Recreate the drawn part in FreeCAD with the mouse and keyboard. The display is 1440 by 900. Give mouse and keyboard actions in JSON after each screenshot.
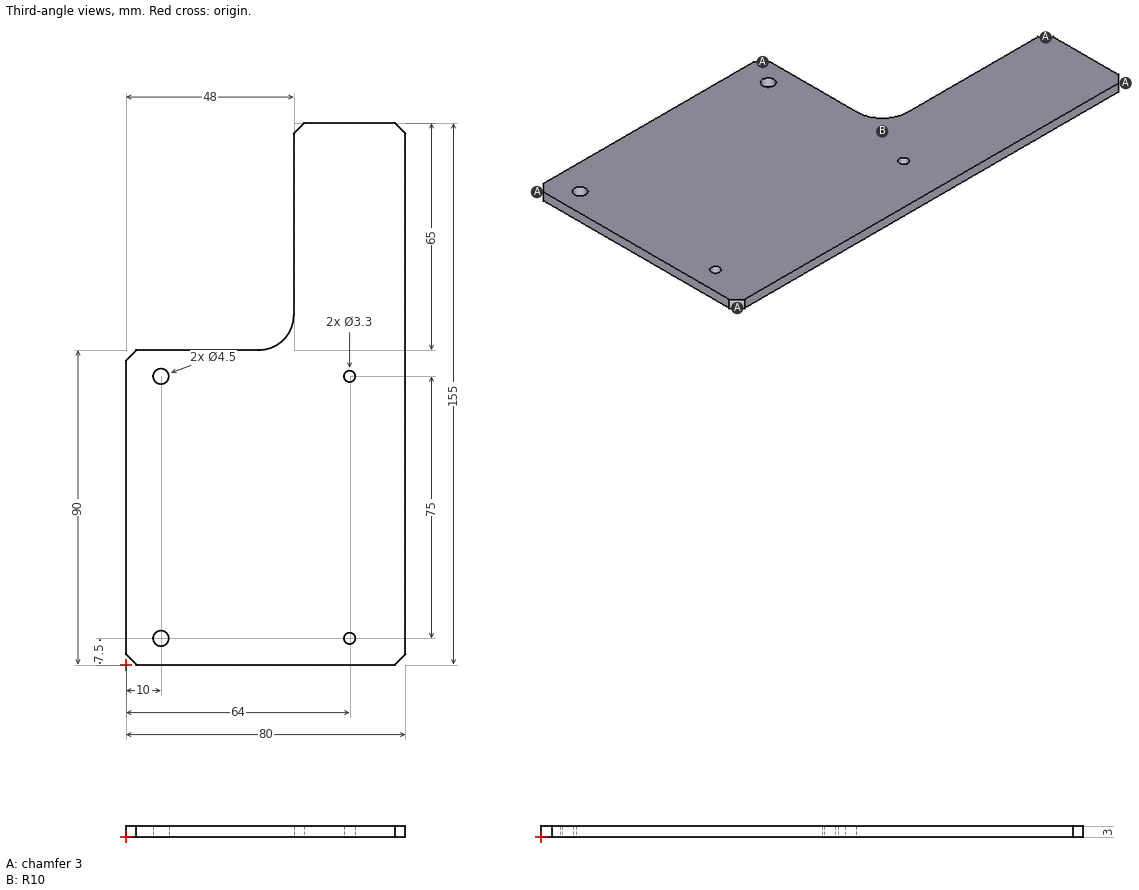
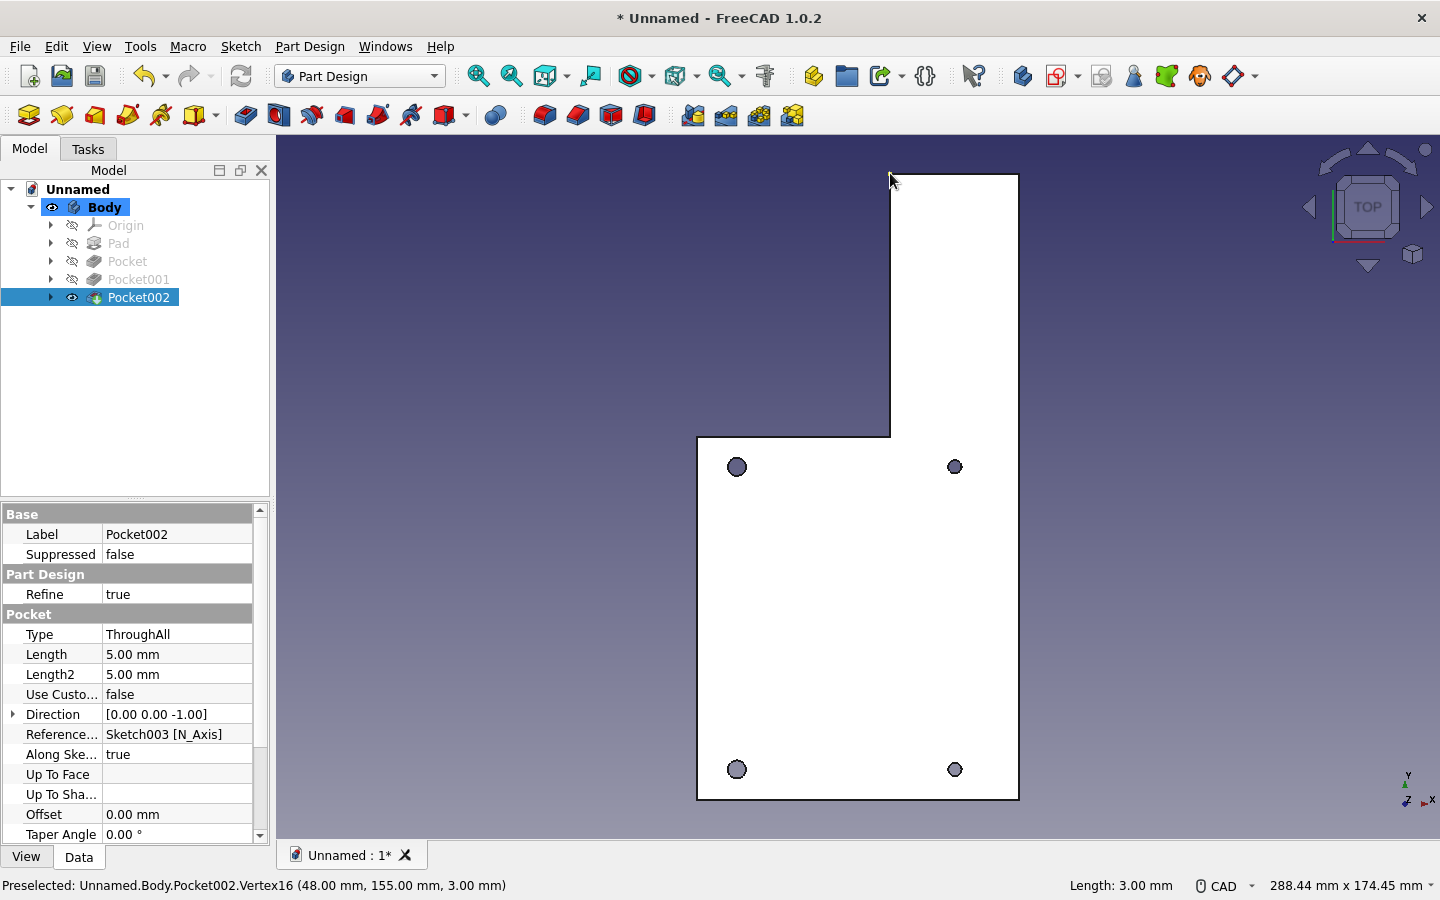
{"action": "key", "text": "1"}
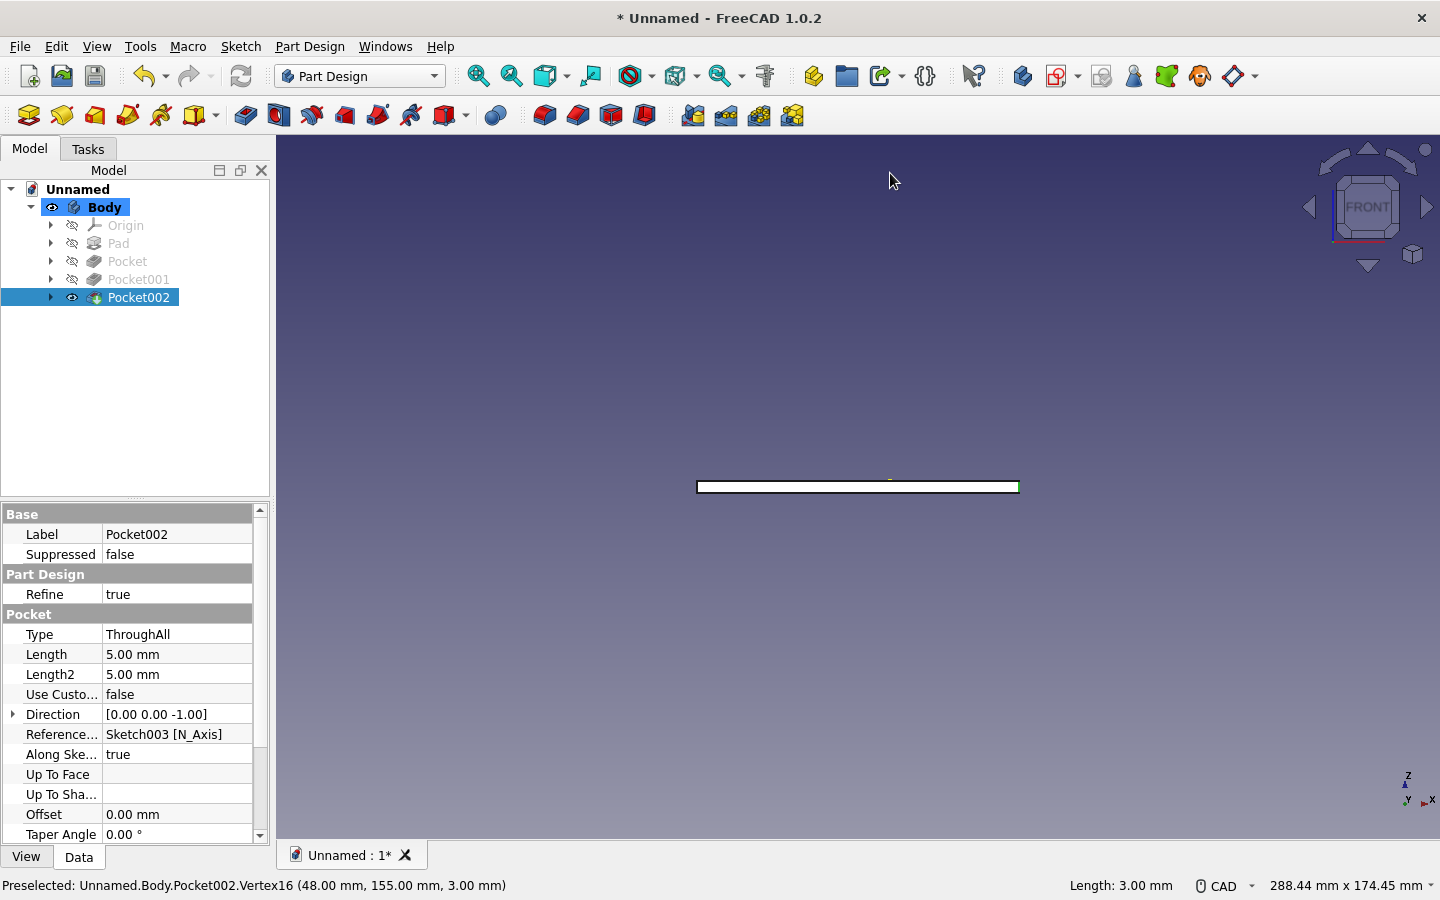
{"action": "key", "text": "v f"}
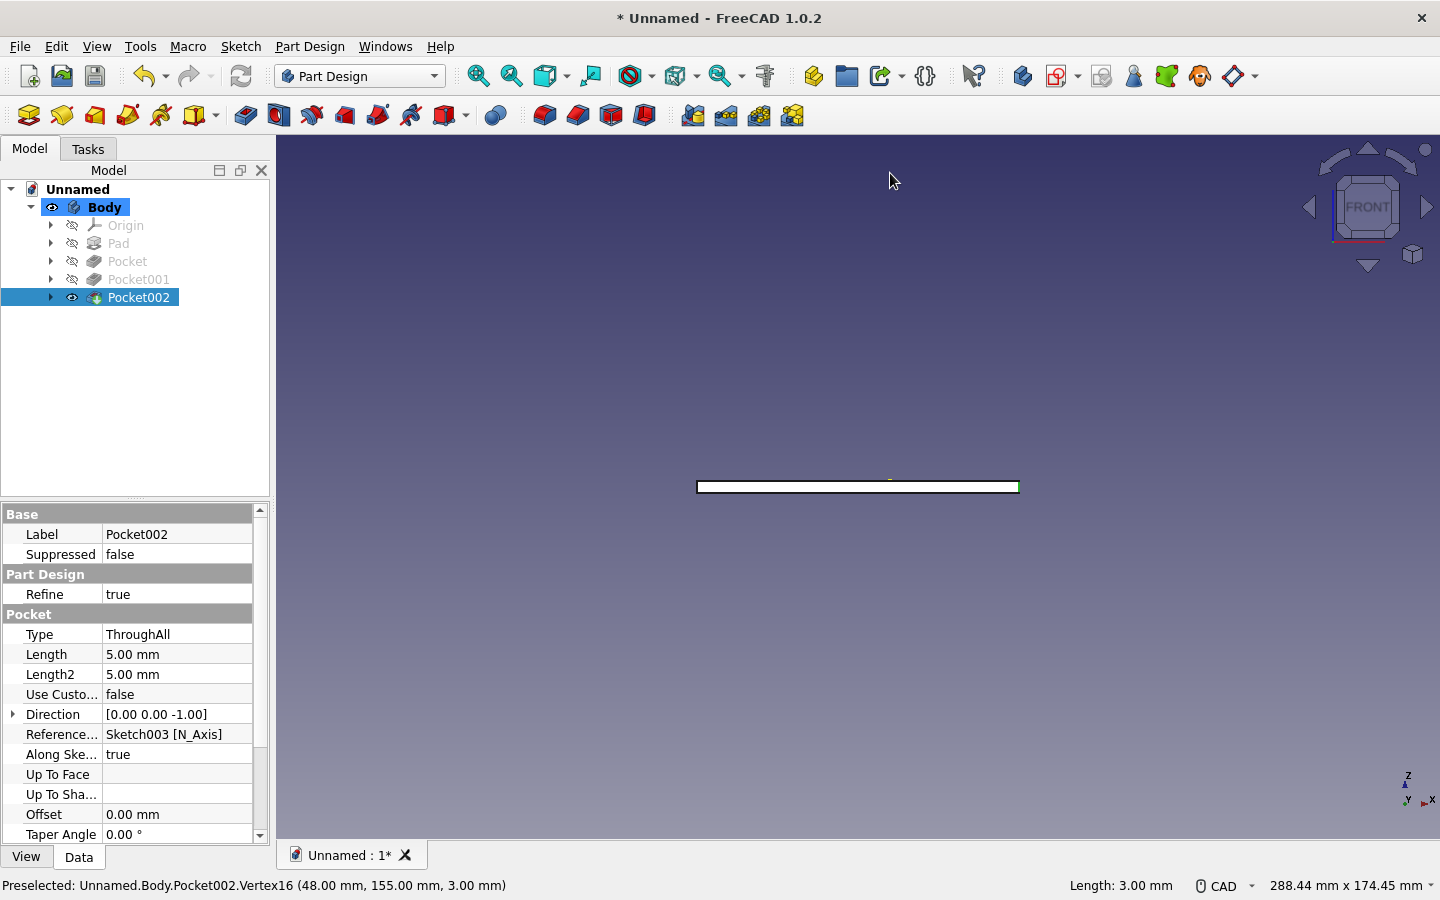
{"action": "left_click", "coordinate": [697, 486], "text": "ctrl"}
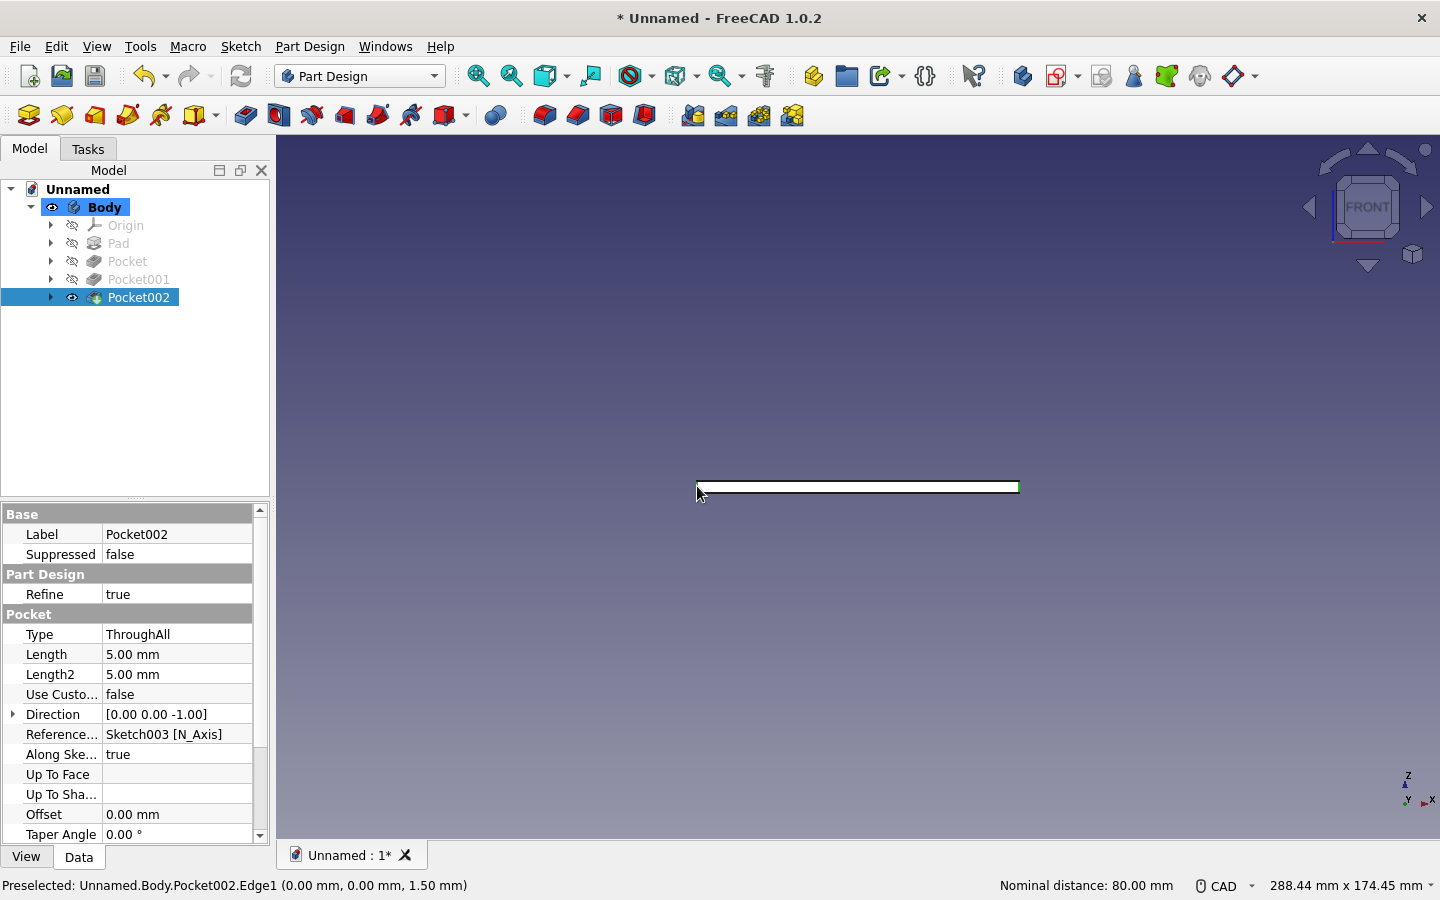
{"action": "scroll", "coordinate": [890, 486], "scroll_direction": "up", "scroll_amount": 6}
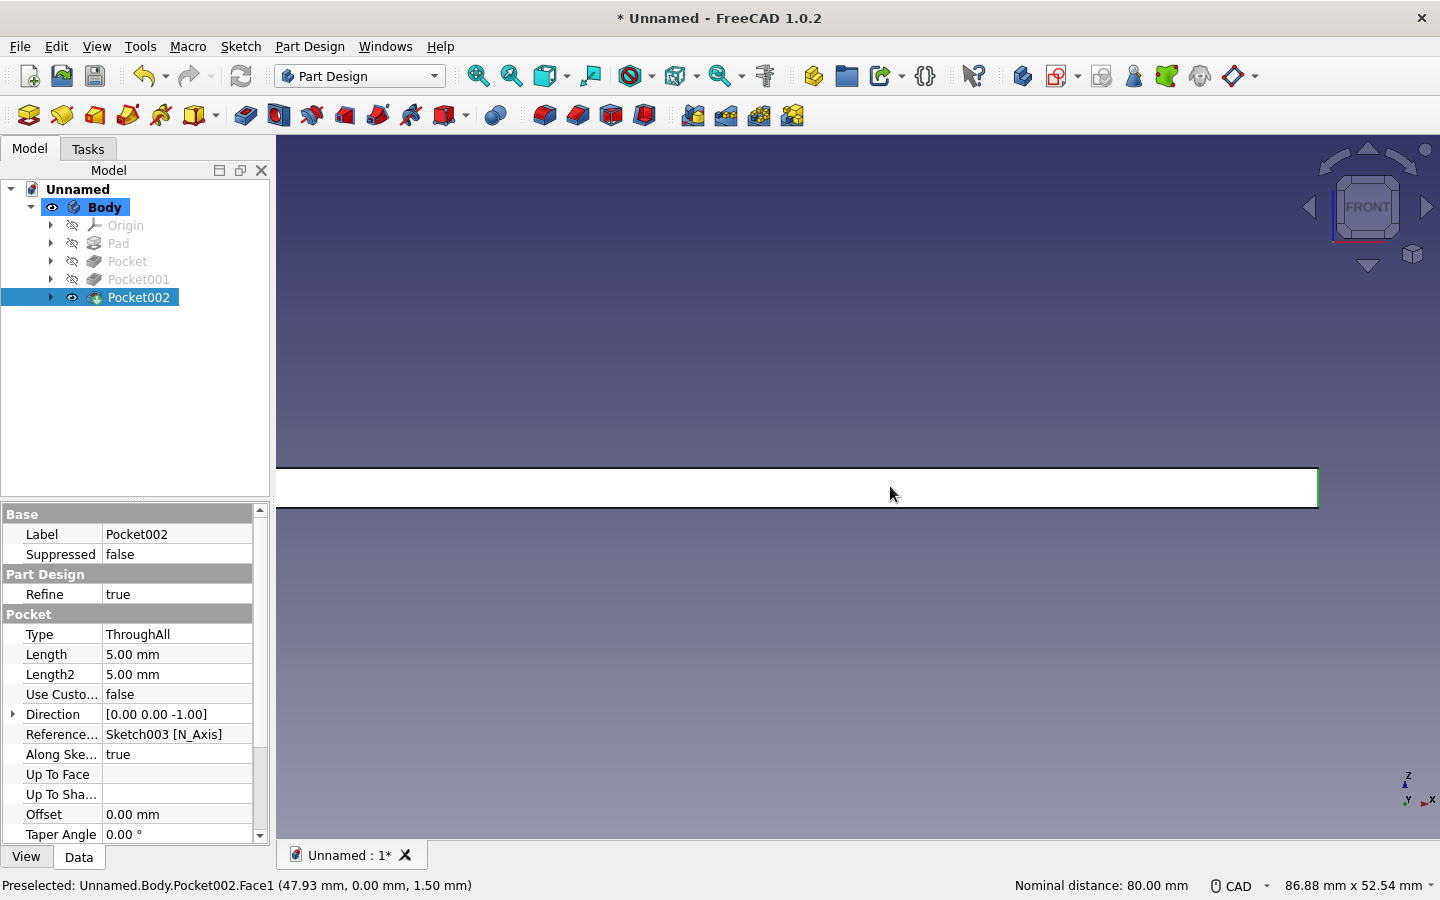
{"action": "key", "text": "v f"}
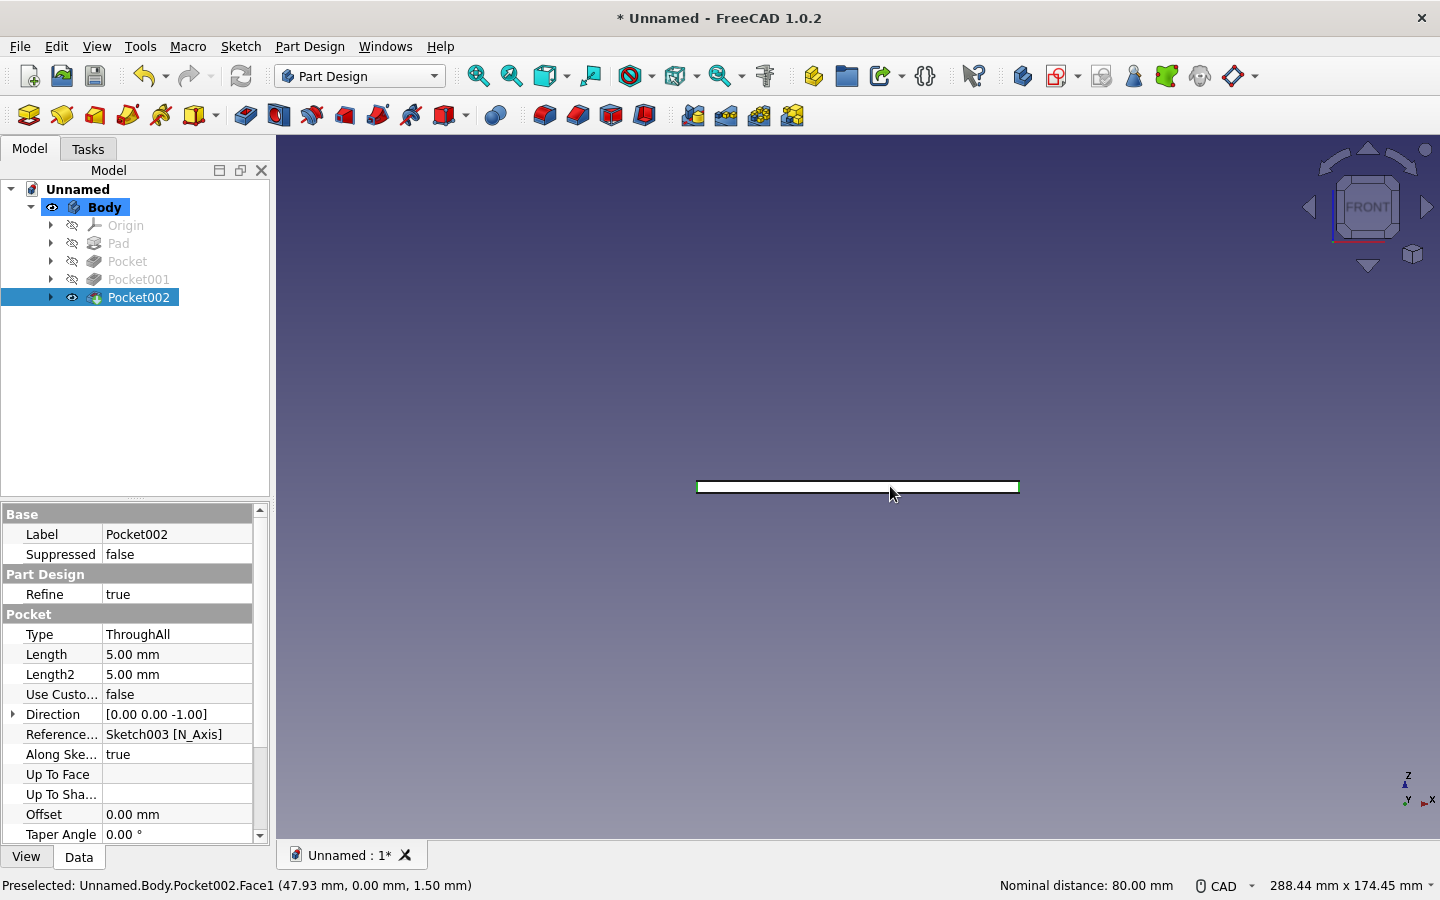
{"action": "key", "text": "3"}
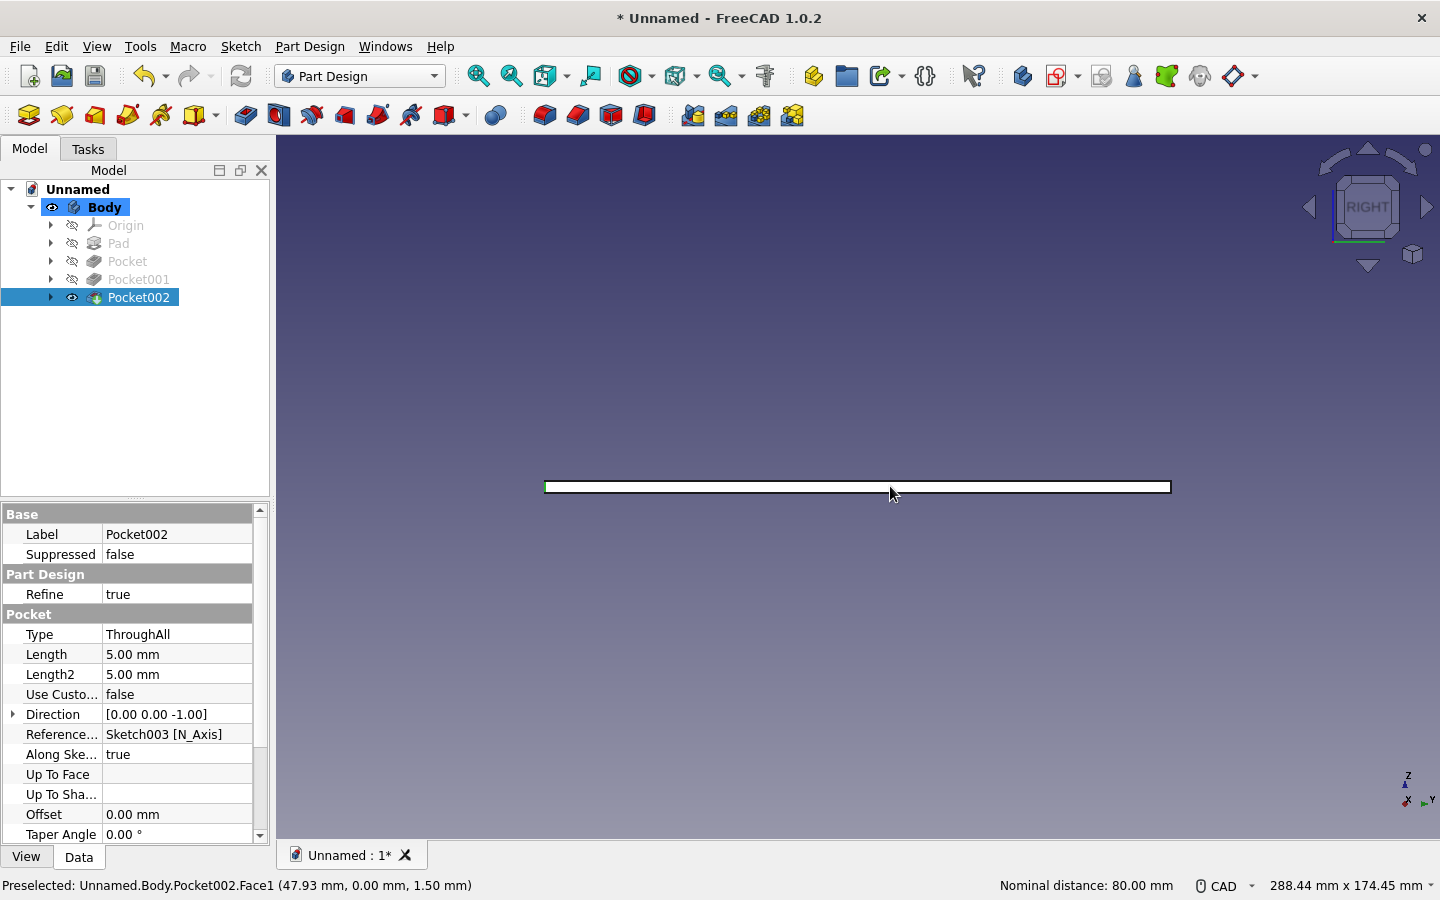
{"action": "left_click", "coordinate": [1171, 486], "text": "ctrl"}